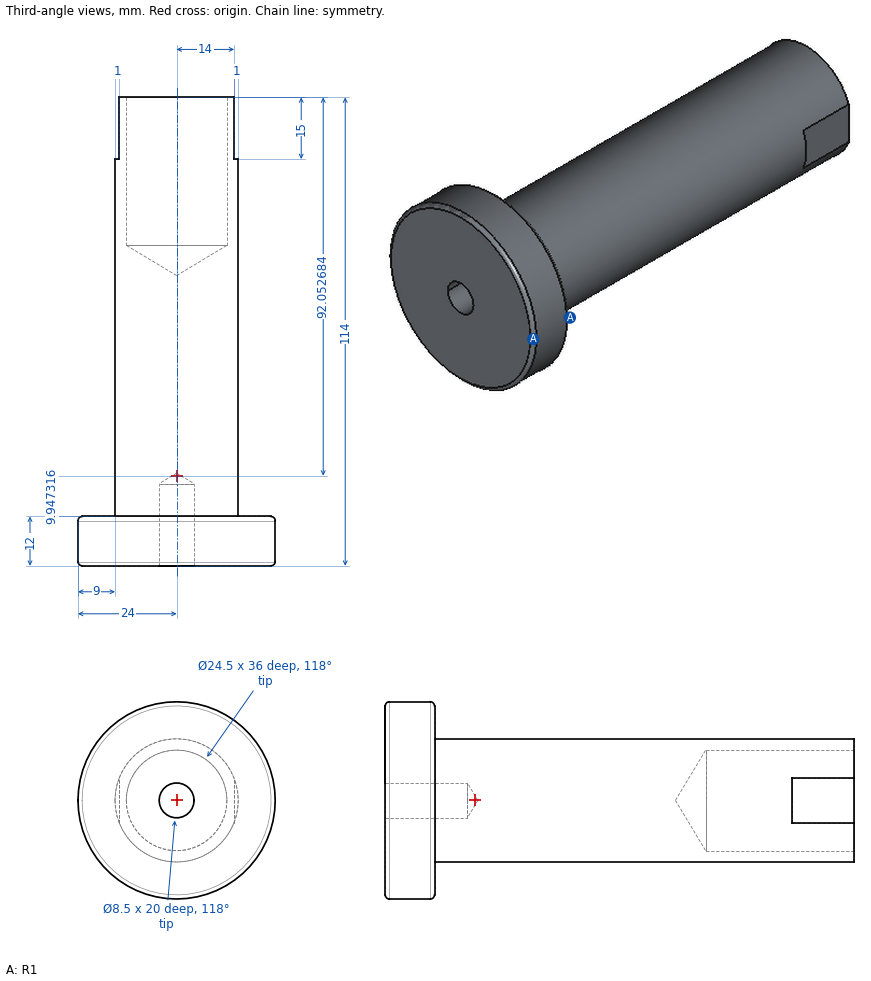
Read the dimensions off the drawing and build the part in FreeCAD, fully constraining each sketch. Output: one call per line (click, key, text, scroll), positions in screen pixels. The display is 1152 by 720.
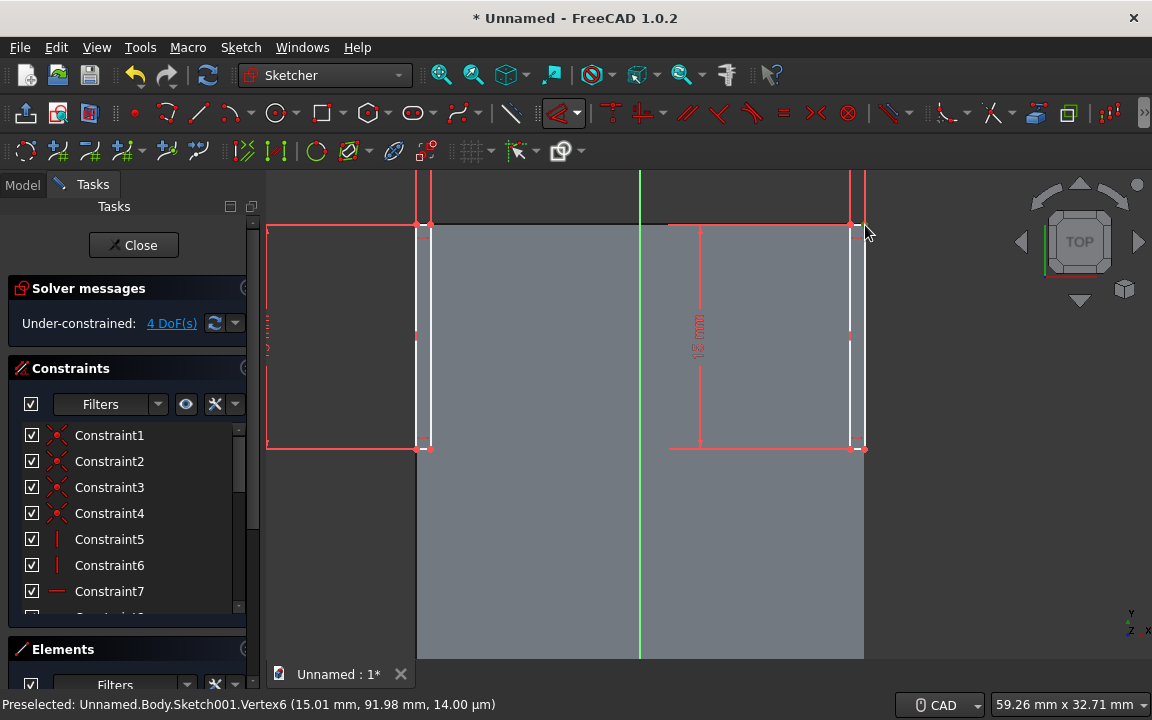
click(416, 225)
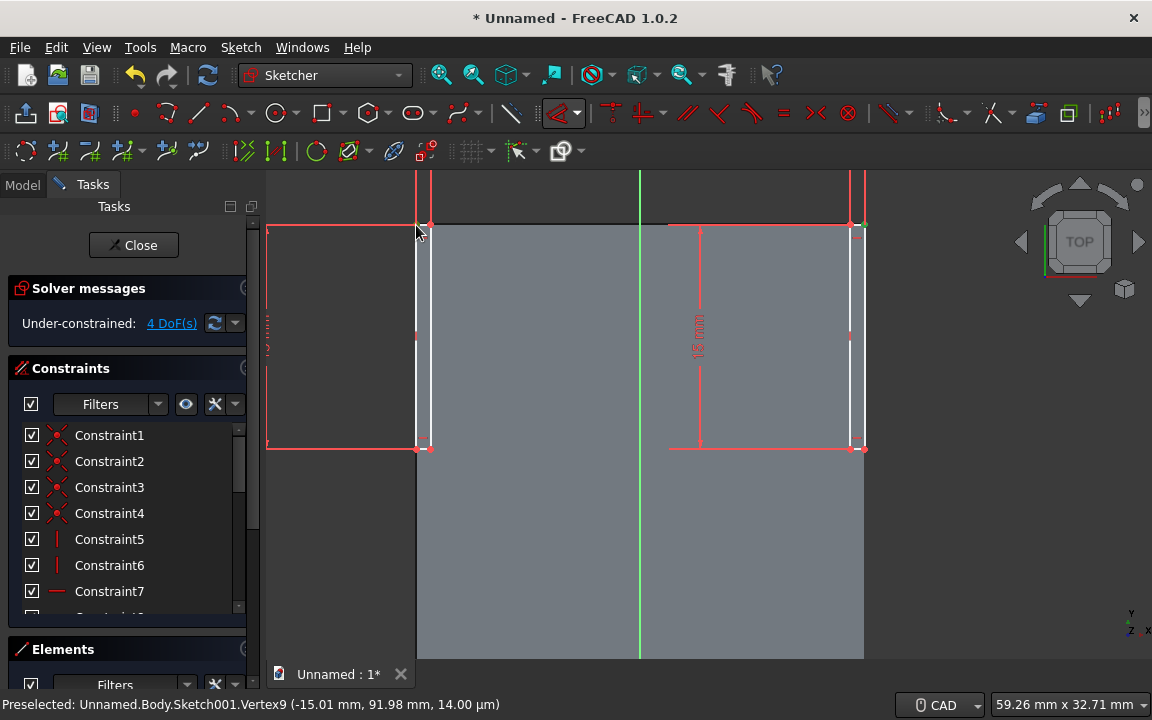
click(640, 600)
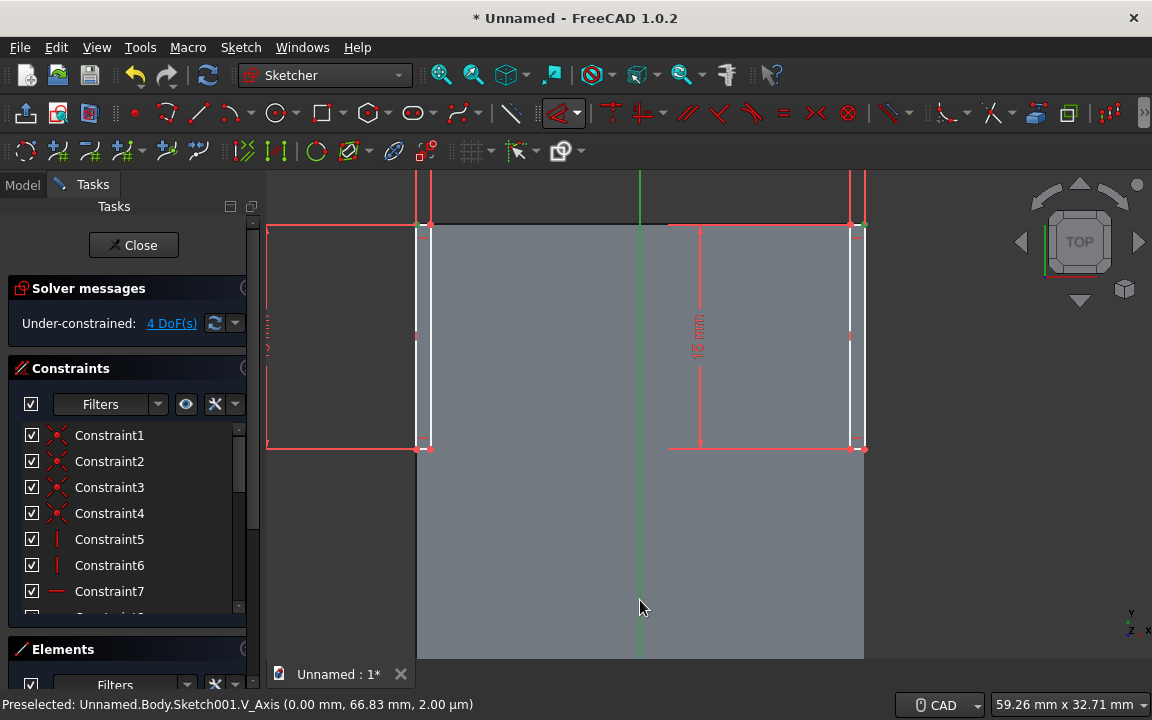
click(816, 114)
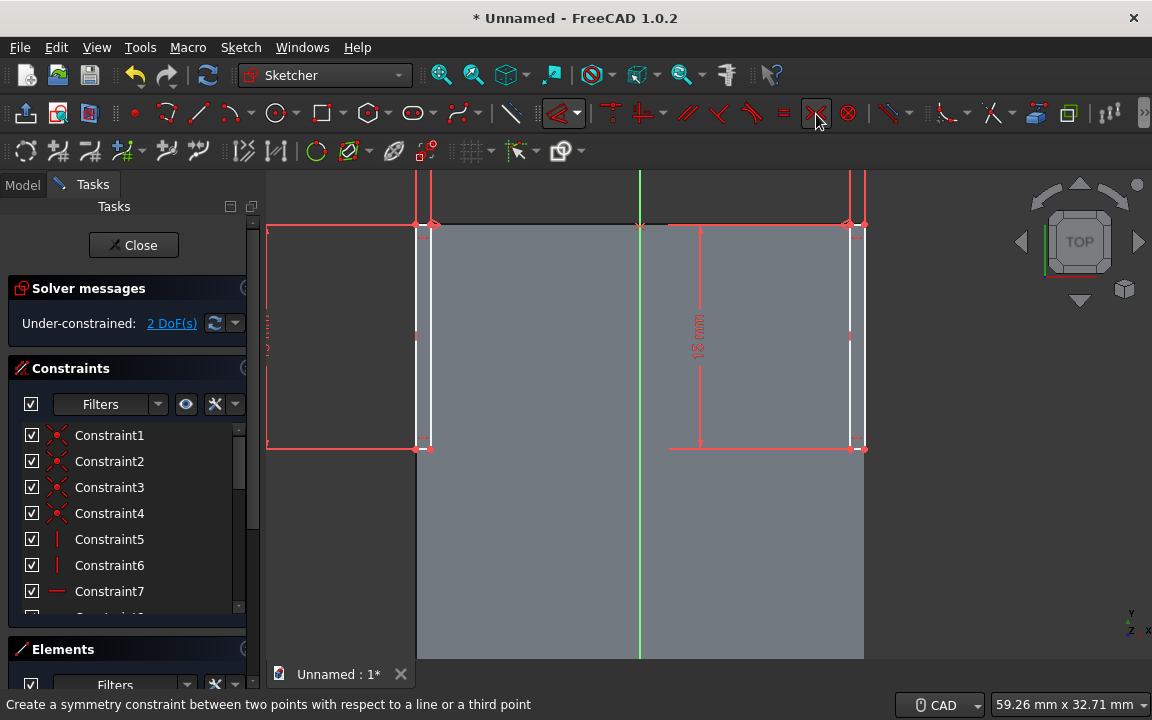
key(d)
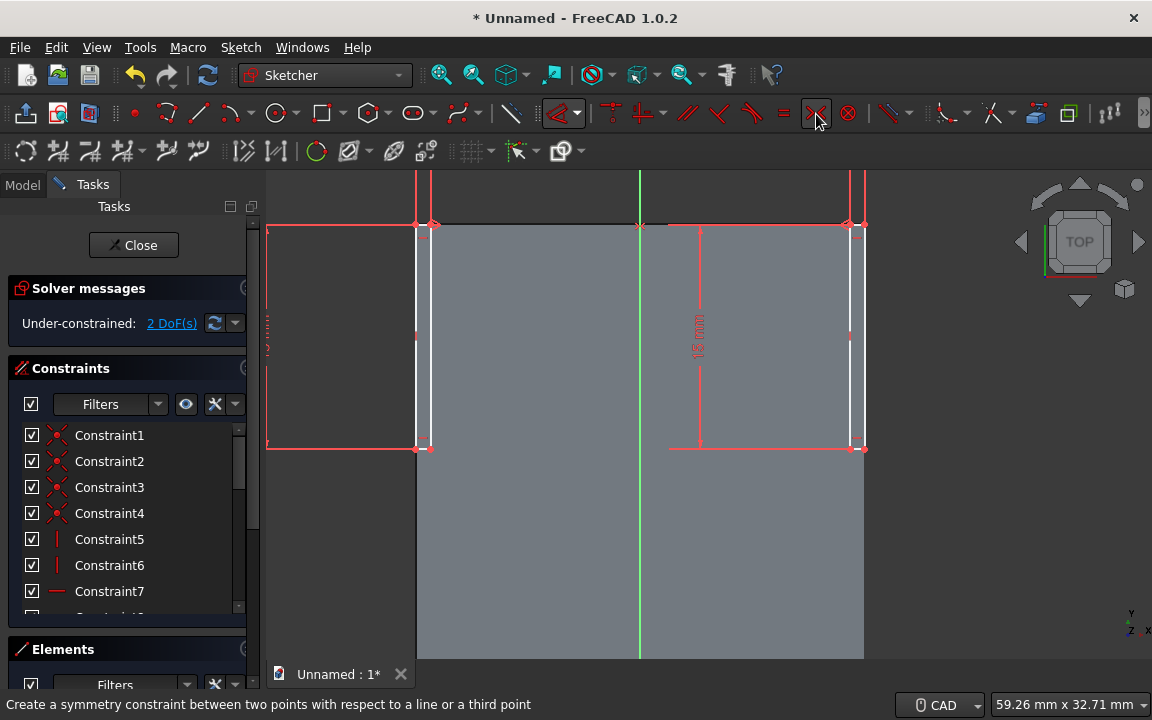
click(850, 225)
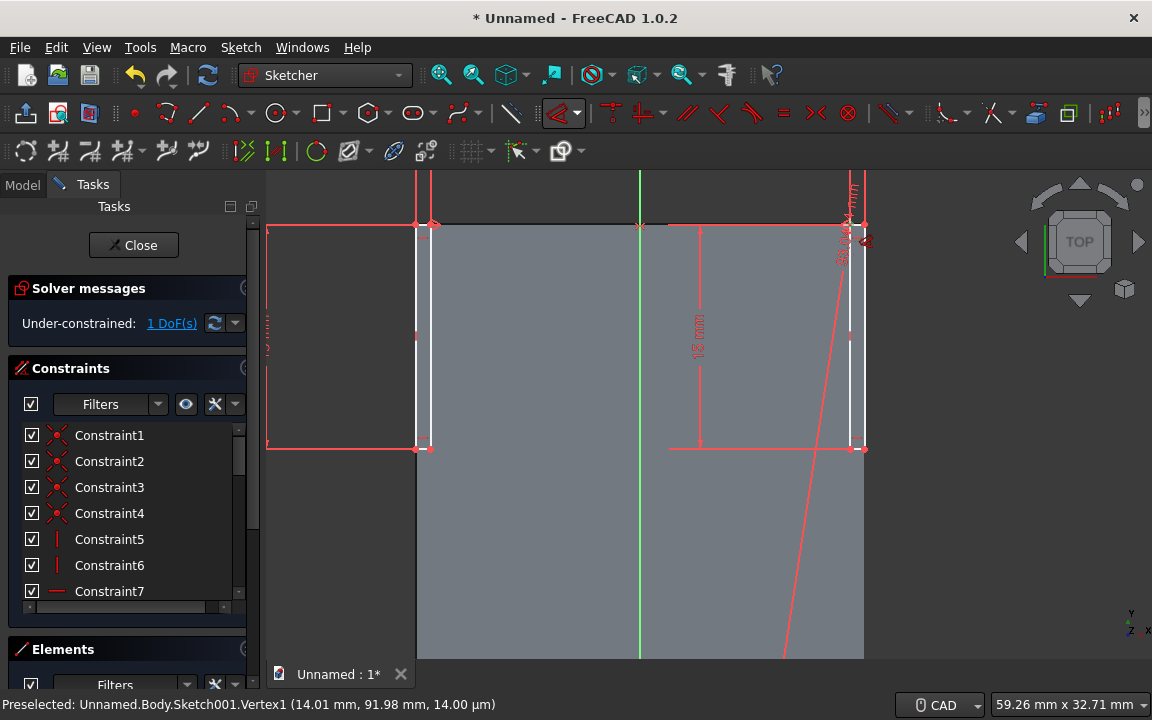
key(Escape)
key(Escape)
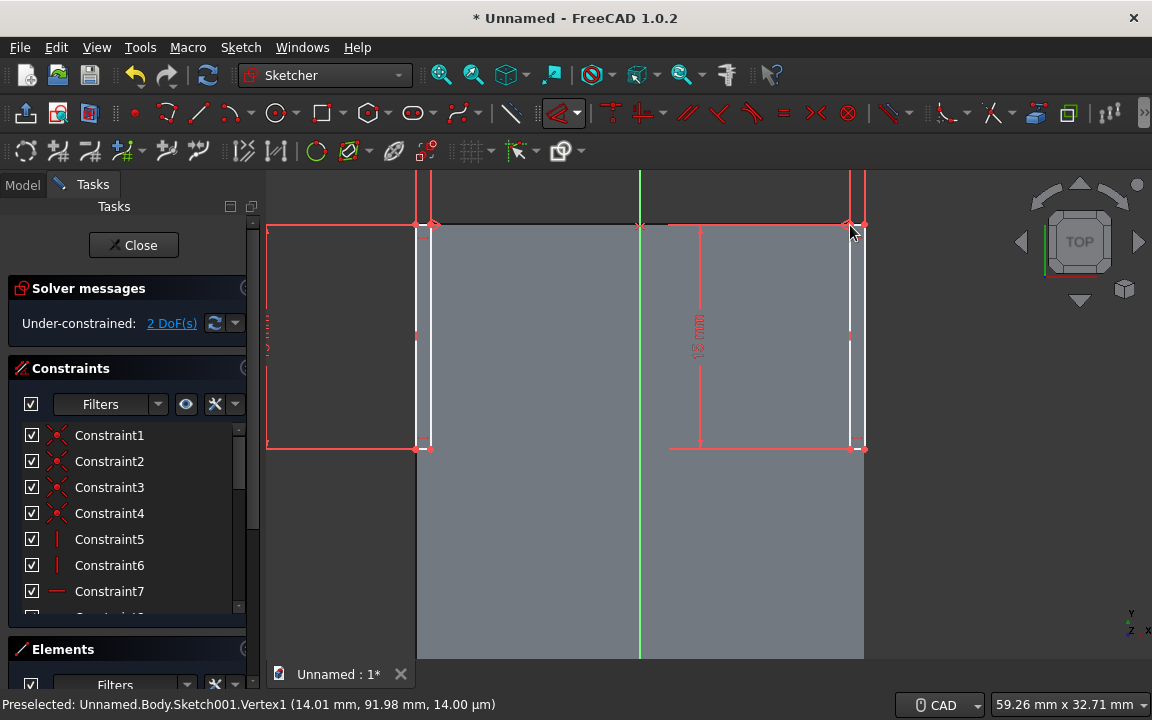
click(850, 225)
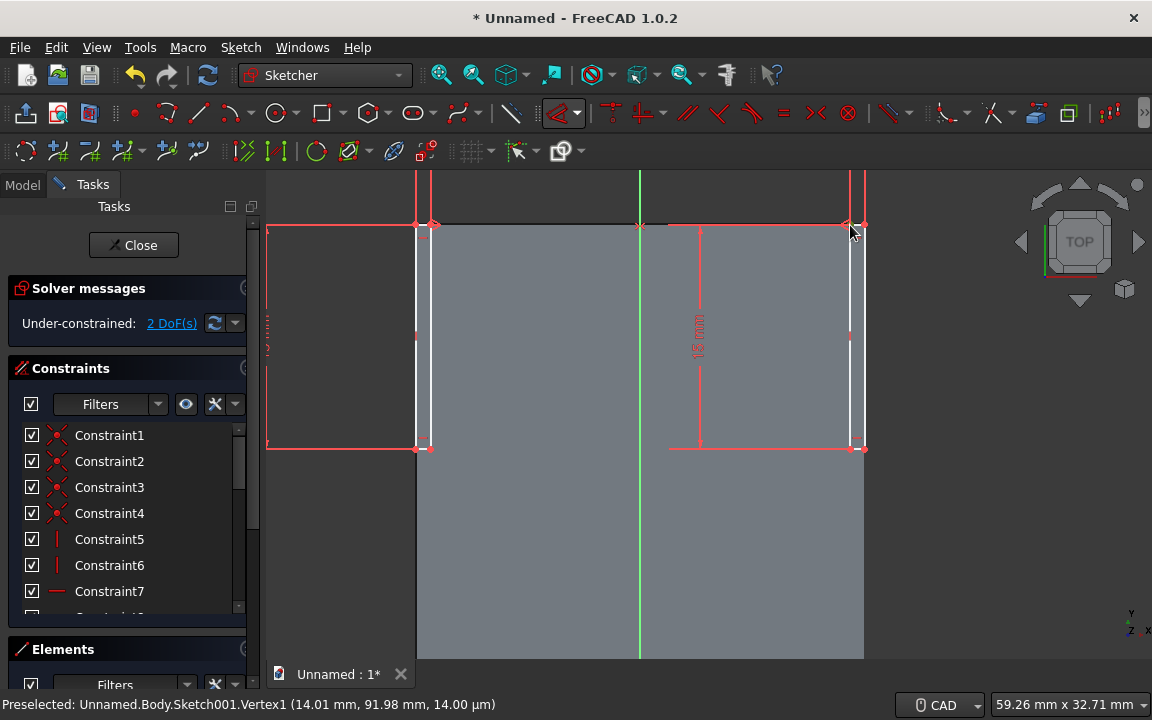
click(580, 114)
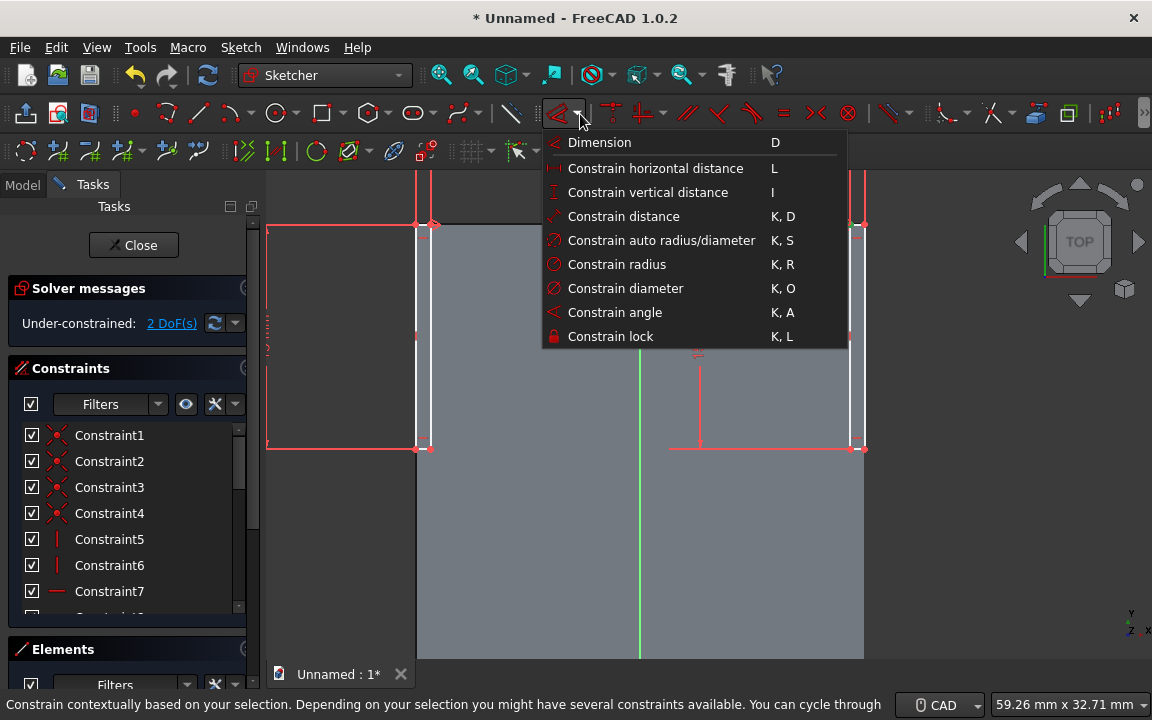
click(695, 168)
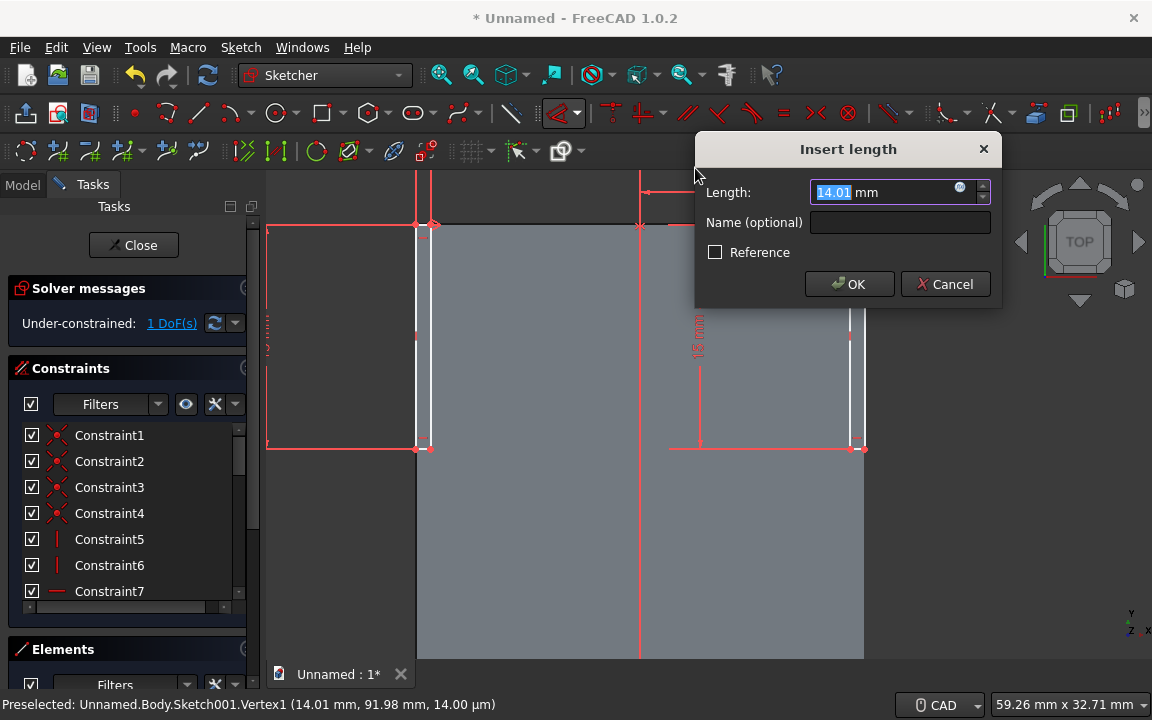
text(14)
key(Return)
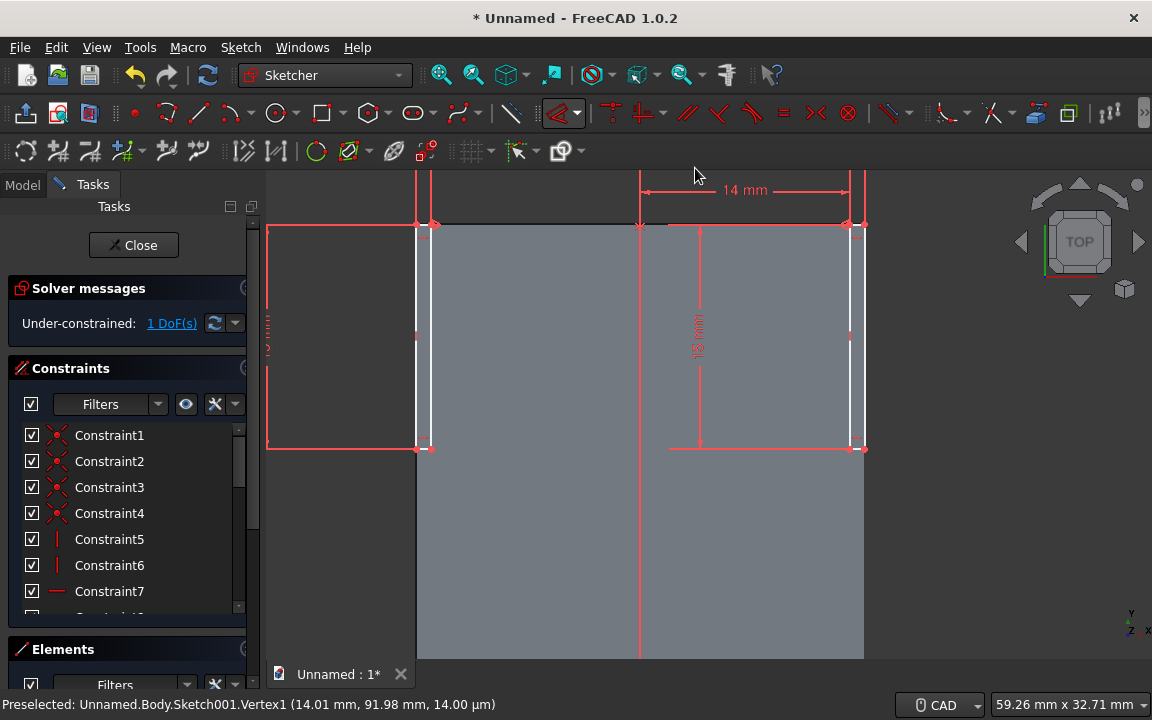
click(850, 225)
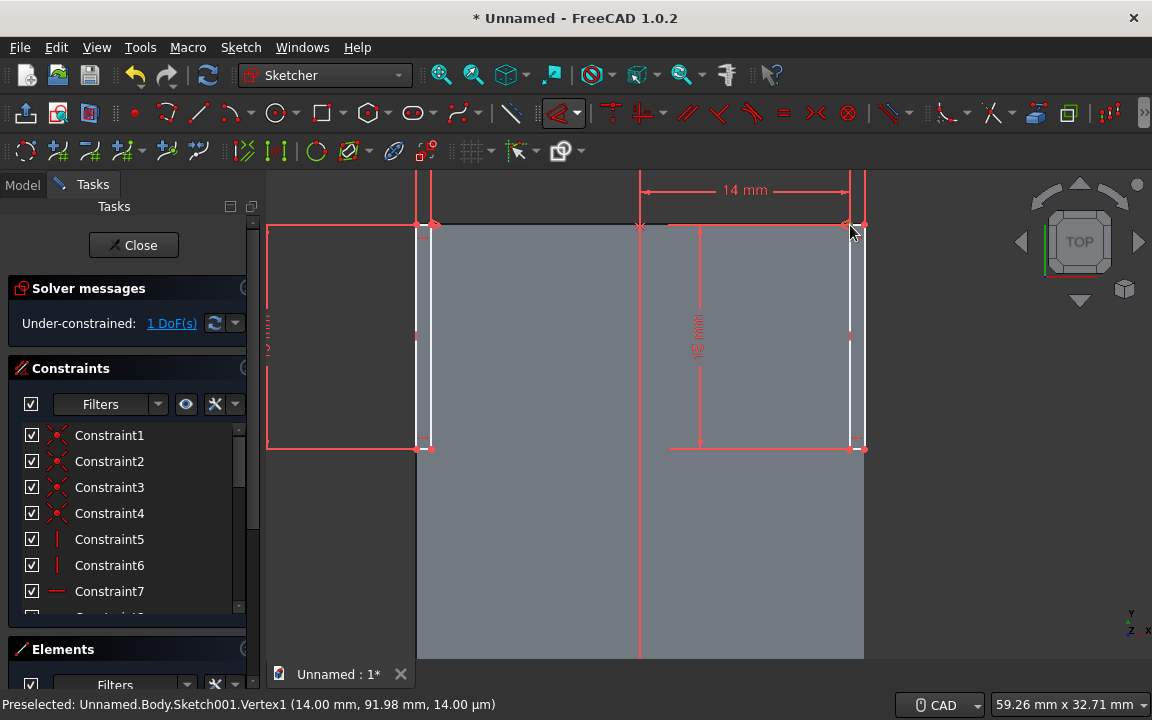
key(i)